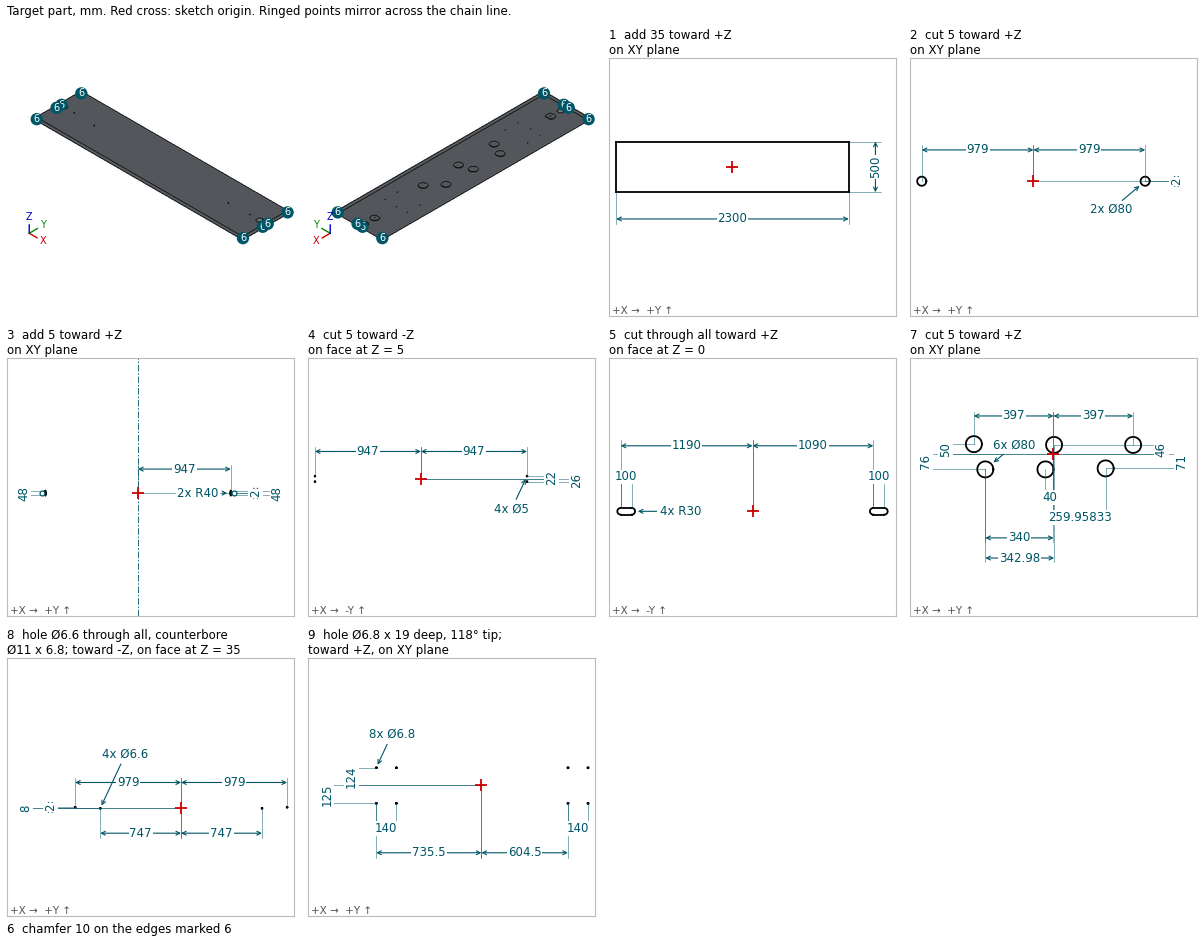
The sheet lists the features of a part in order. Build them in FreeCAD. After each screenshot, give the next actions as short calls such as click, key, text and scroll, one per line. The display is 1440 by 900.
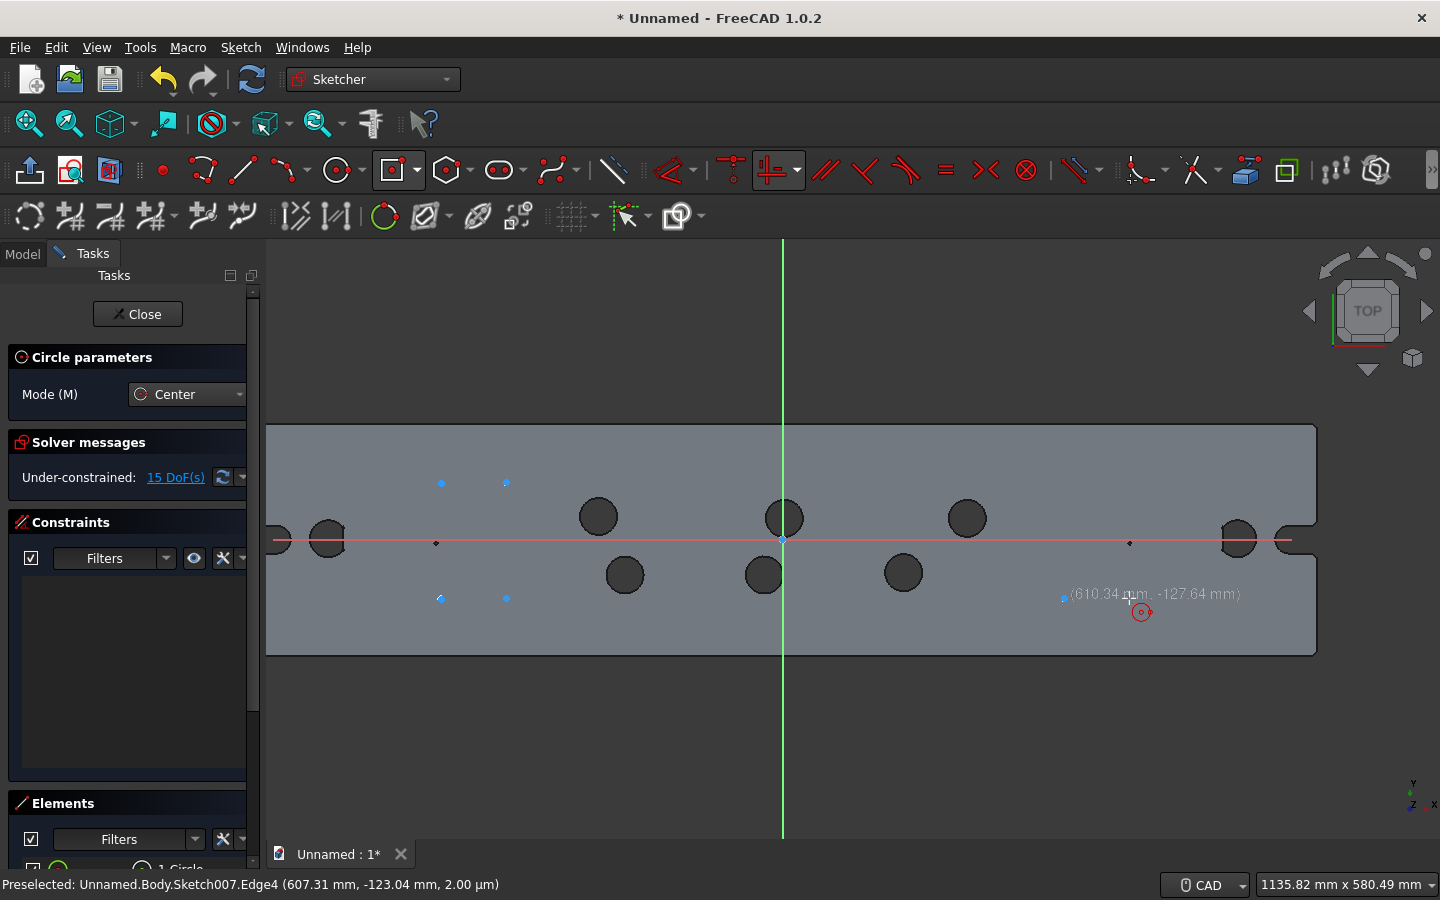
click(1129, 598)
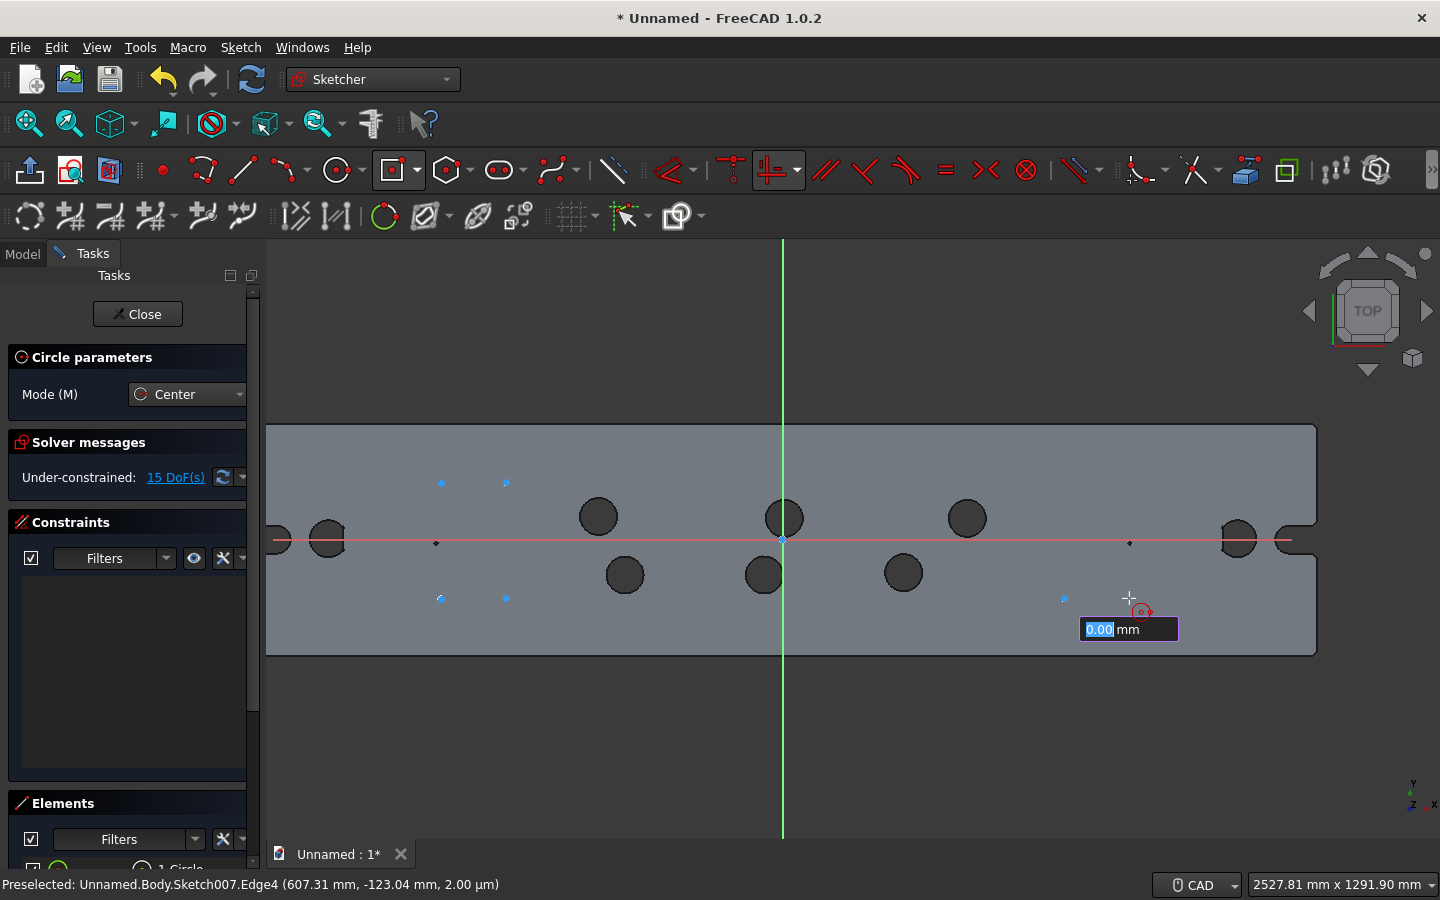
scroll(1130, 597, up, 12)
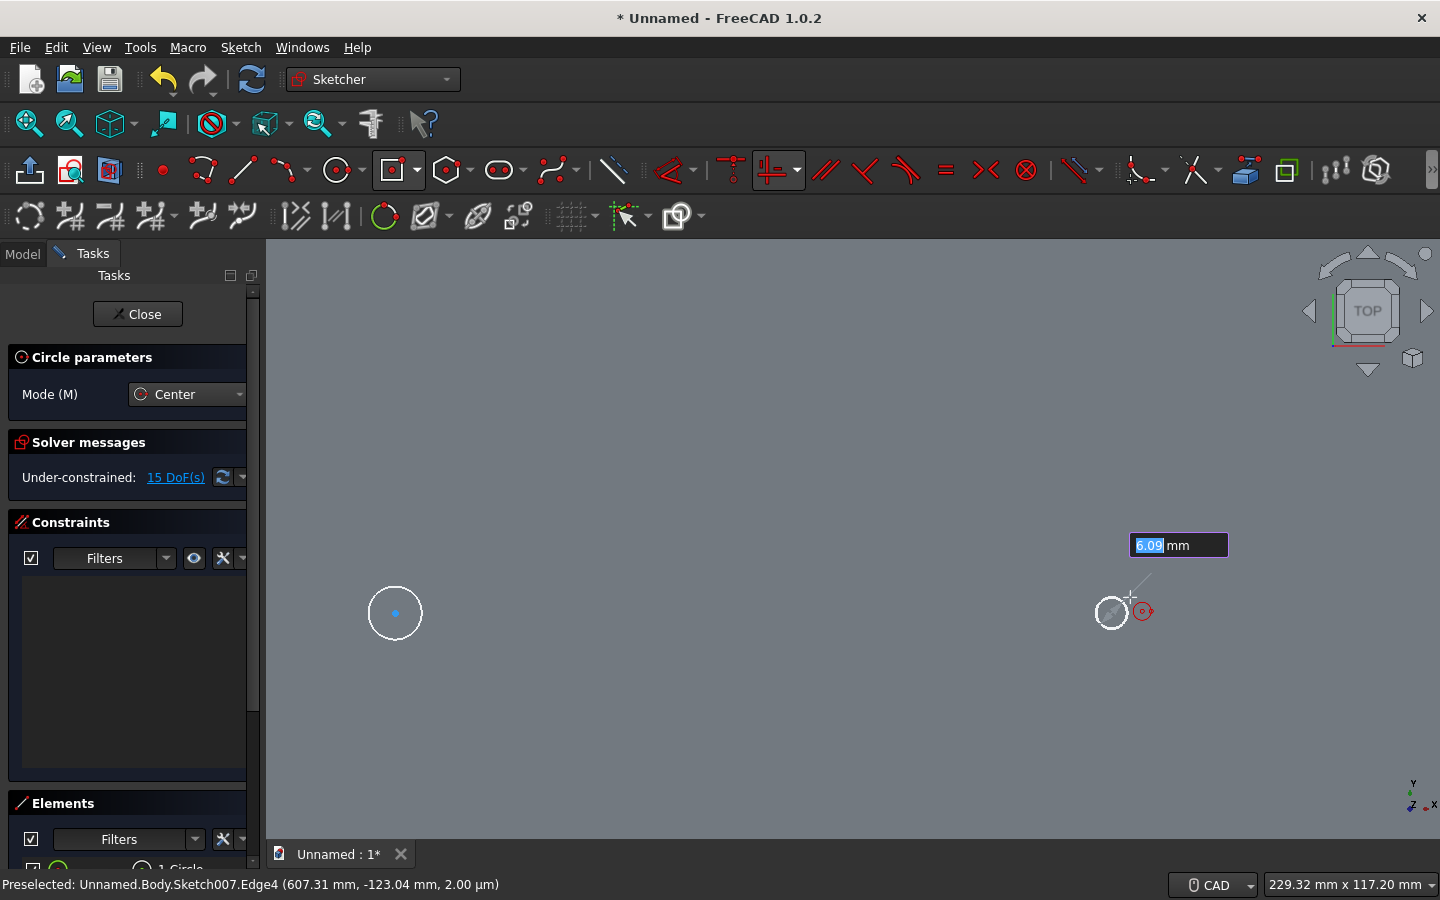
click(1121, 587)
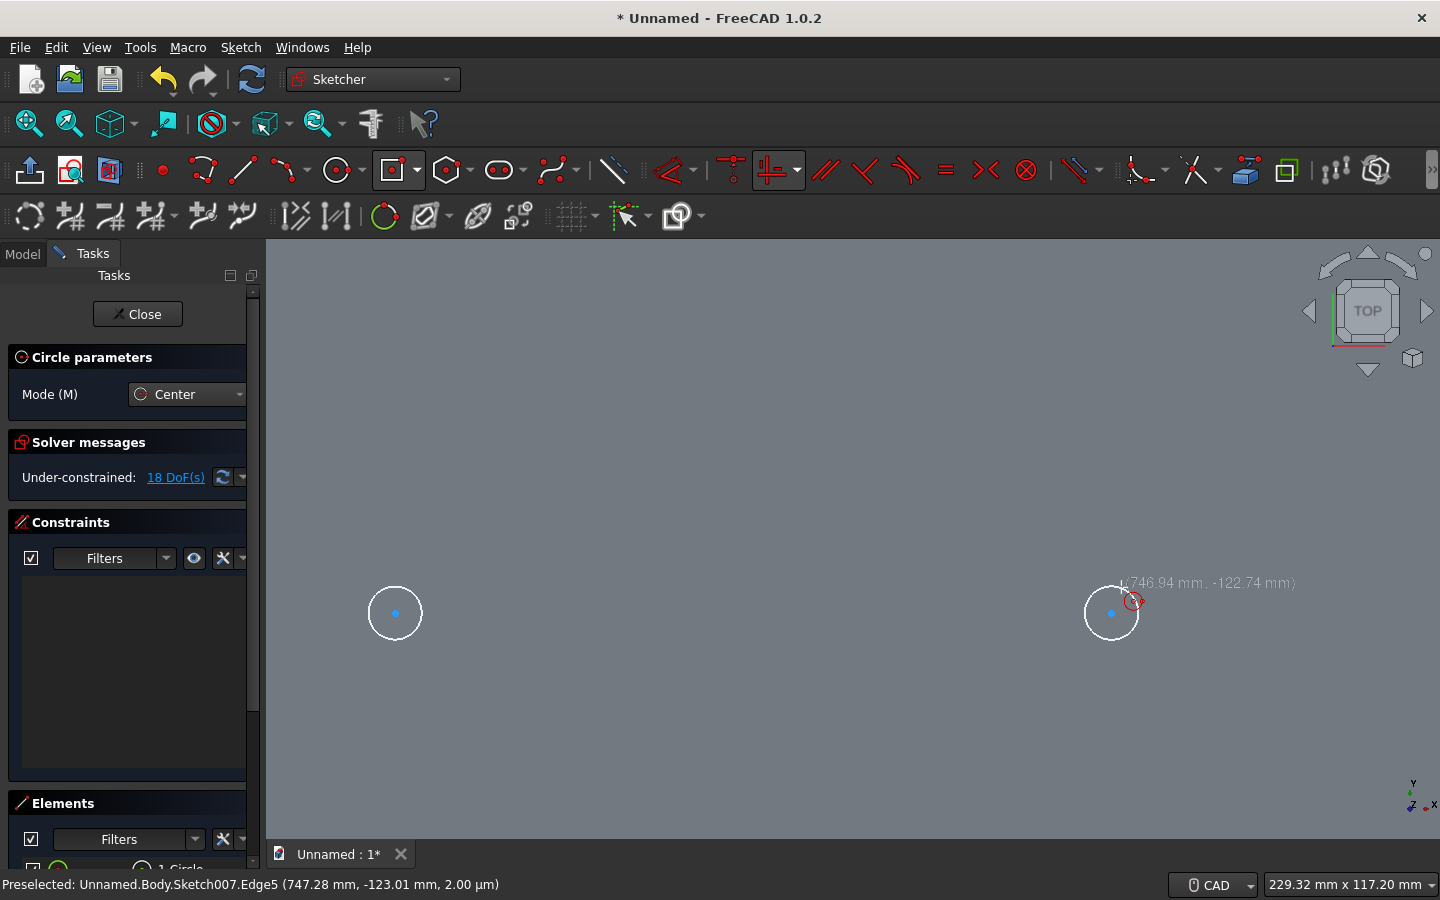
scroll(1130, 597, down, 12)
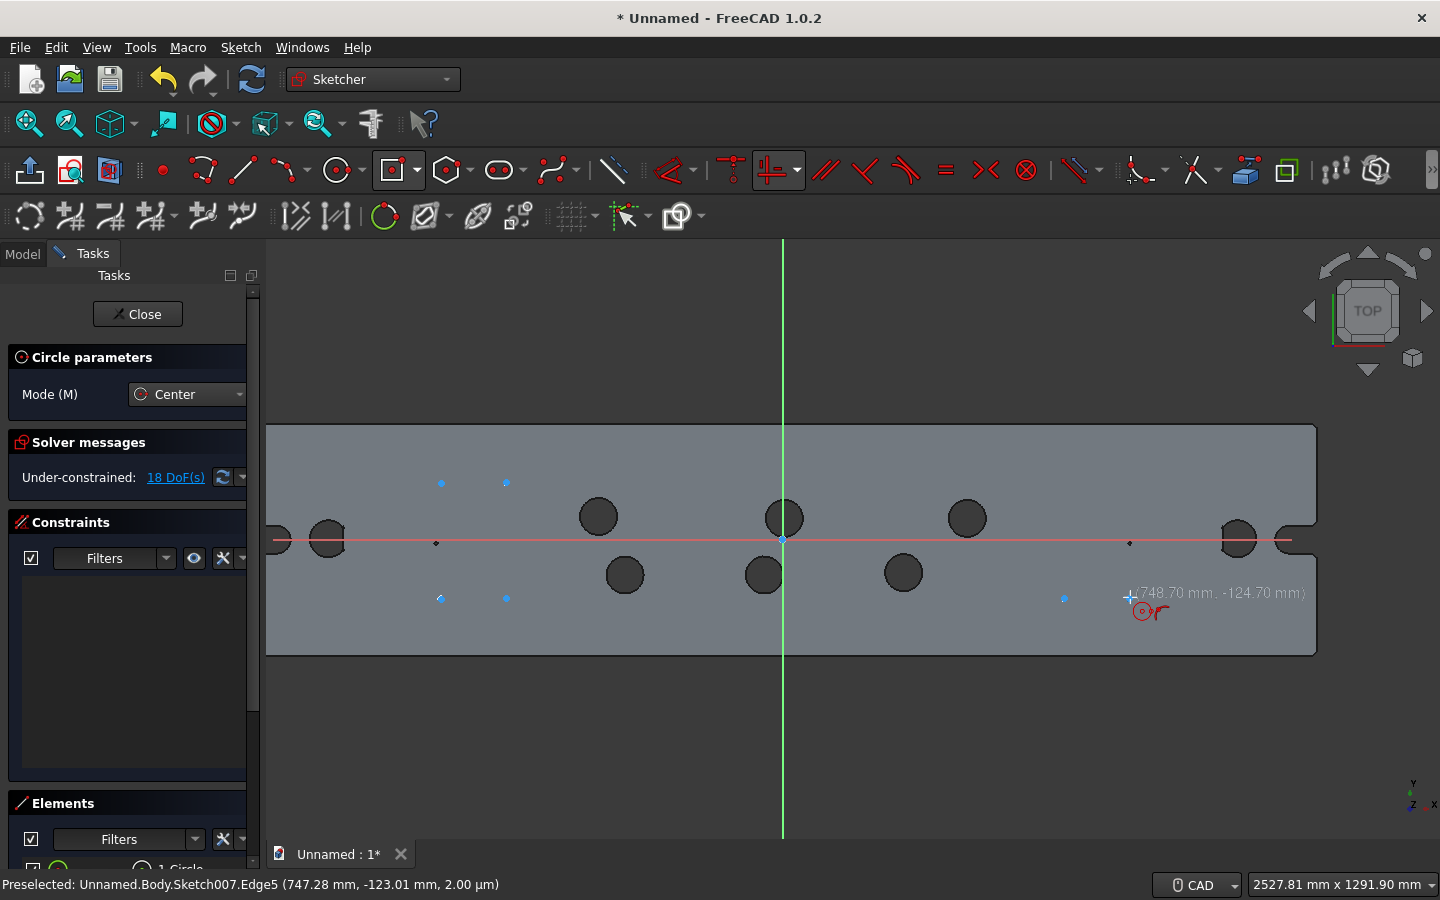
scroll(1064, 482, up, 14)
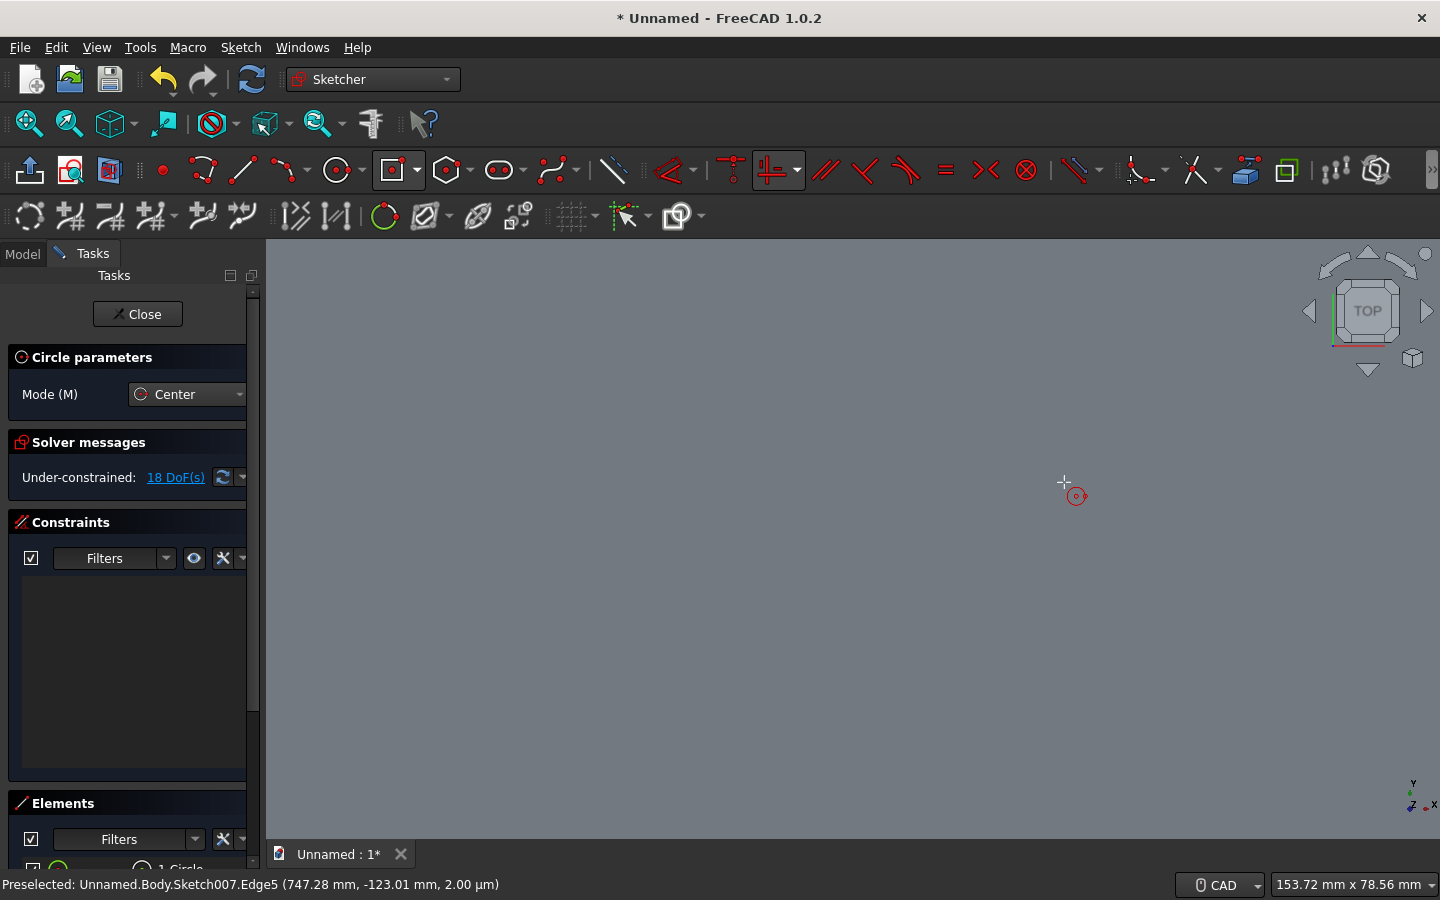
scroll(1064, 481, down, 14)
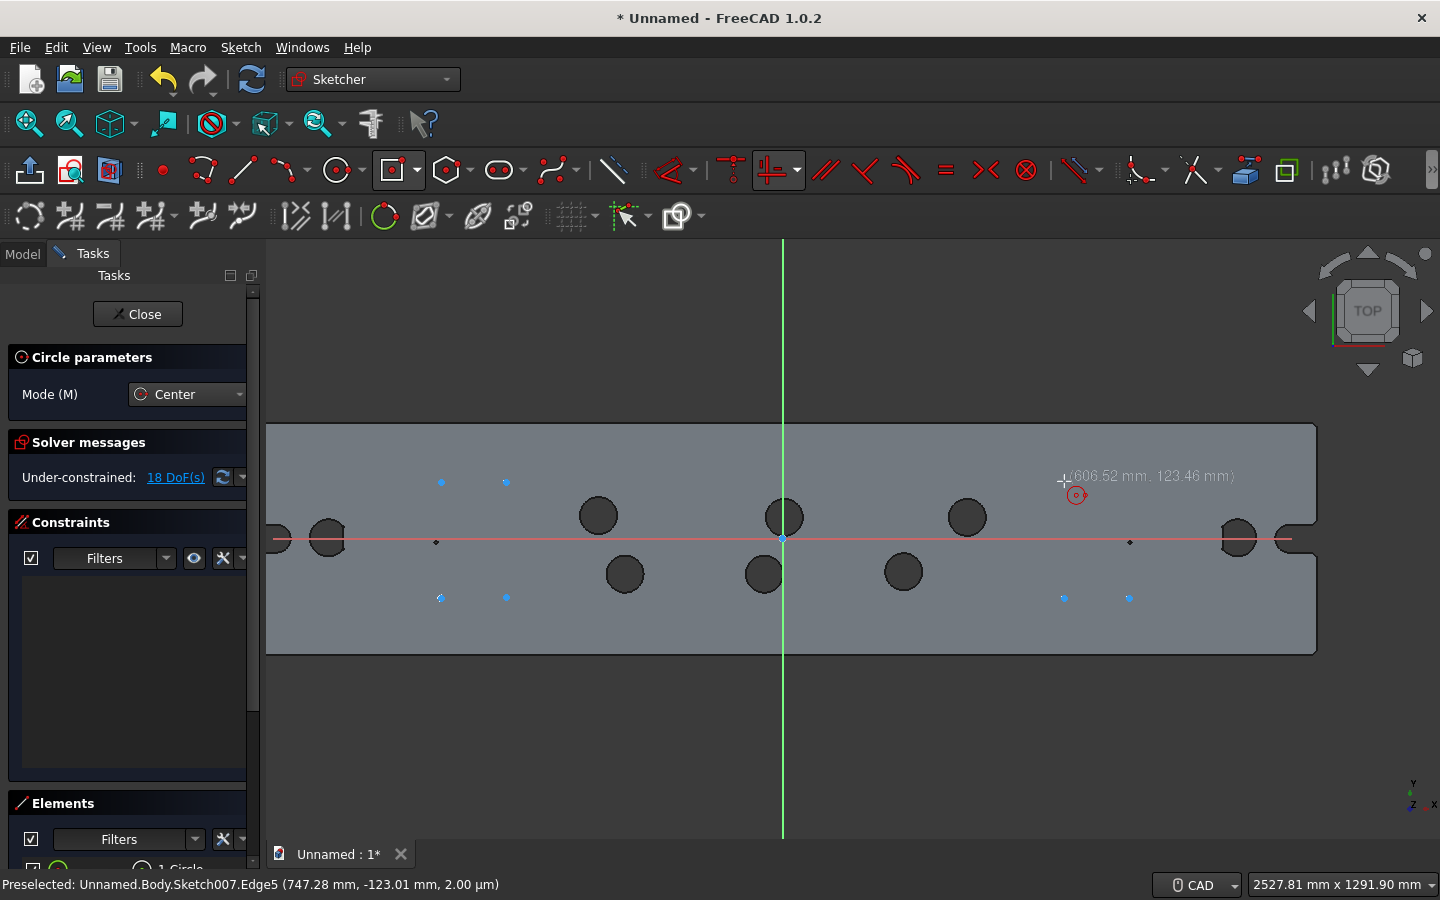
click(1064, 481)